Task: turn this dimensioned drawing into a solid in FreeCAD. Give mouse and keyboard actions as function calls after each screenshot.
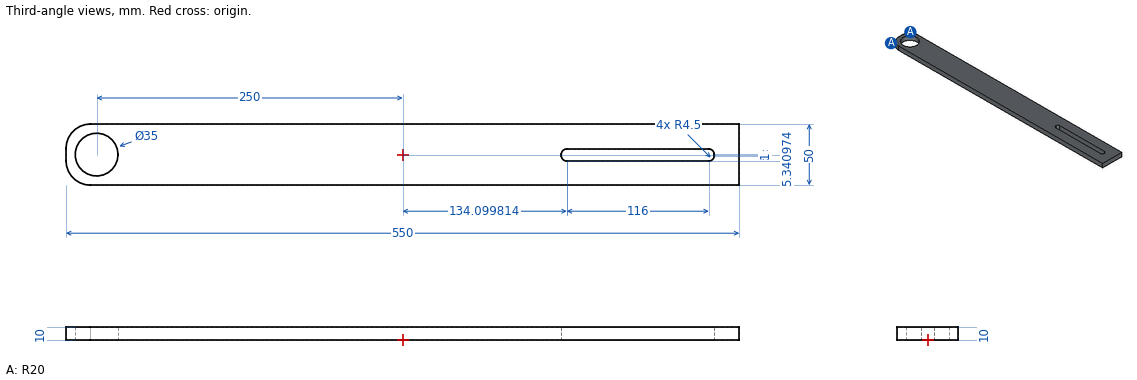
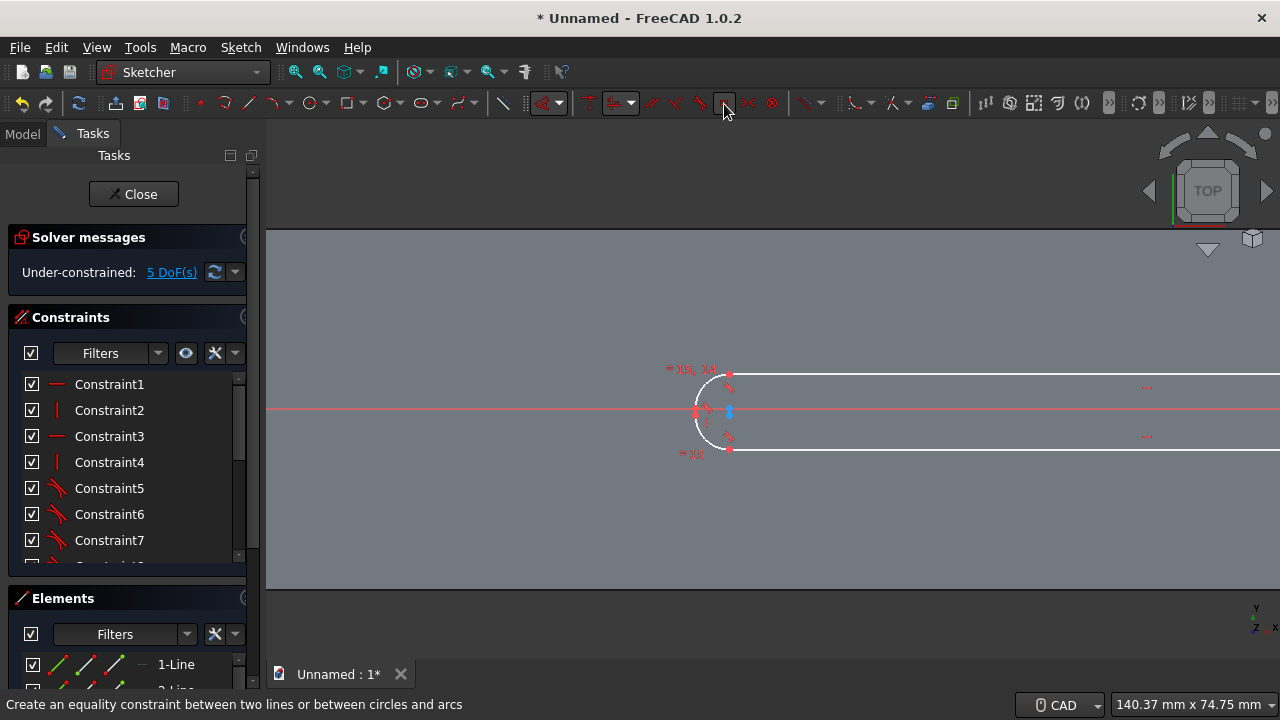
scroll(715, 379, down, 6)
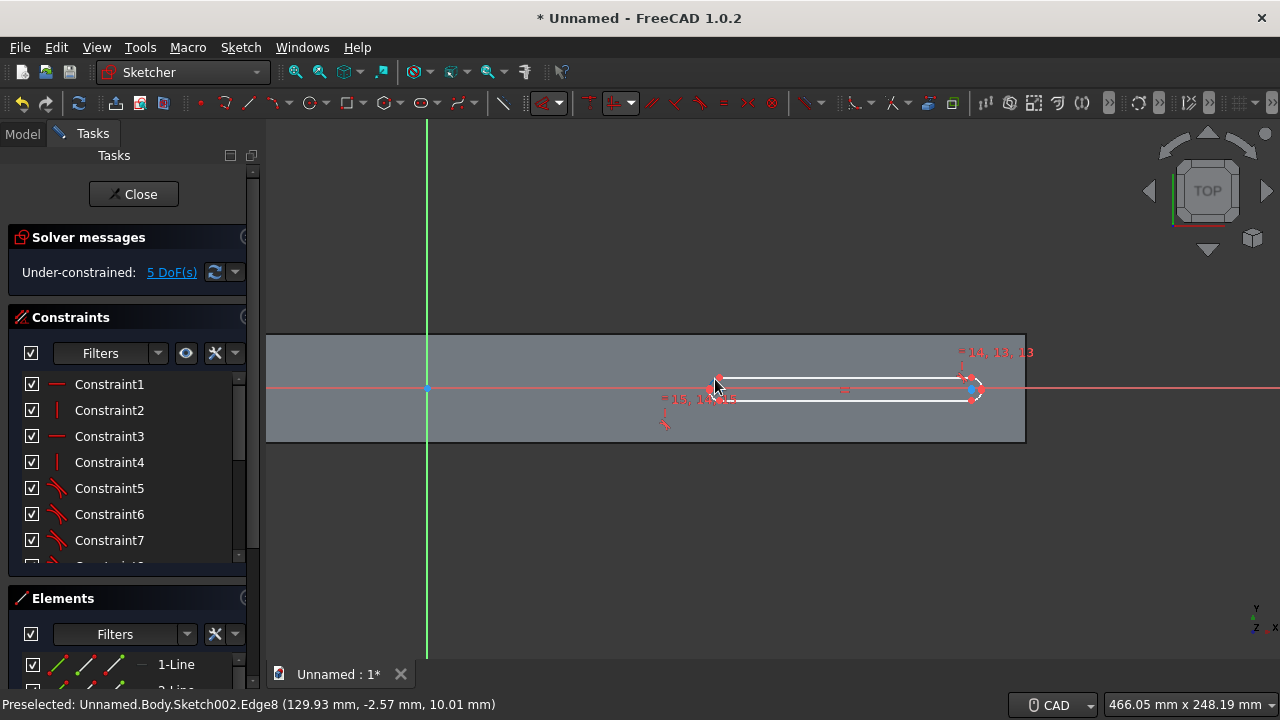
scroll(976, 400, up, 7)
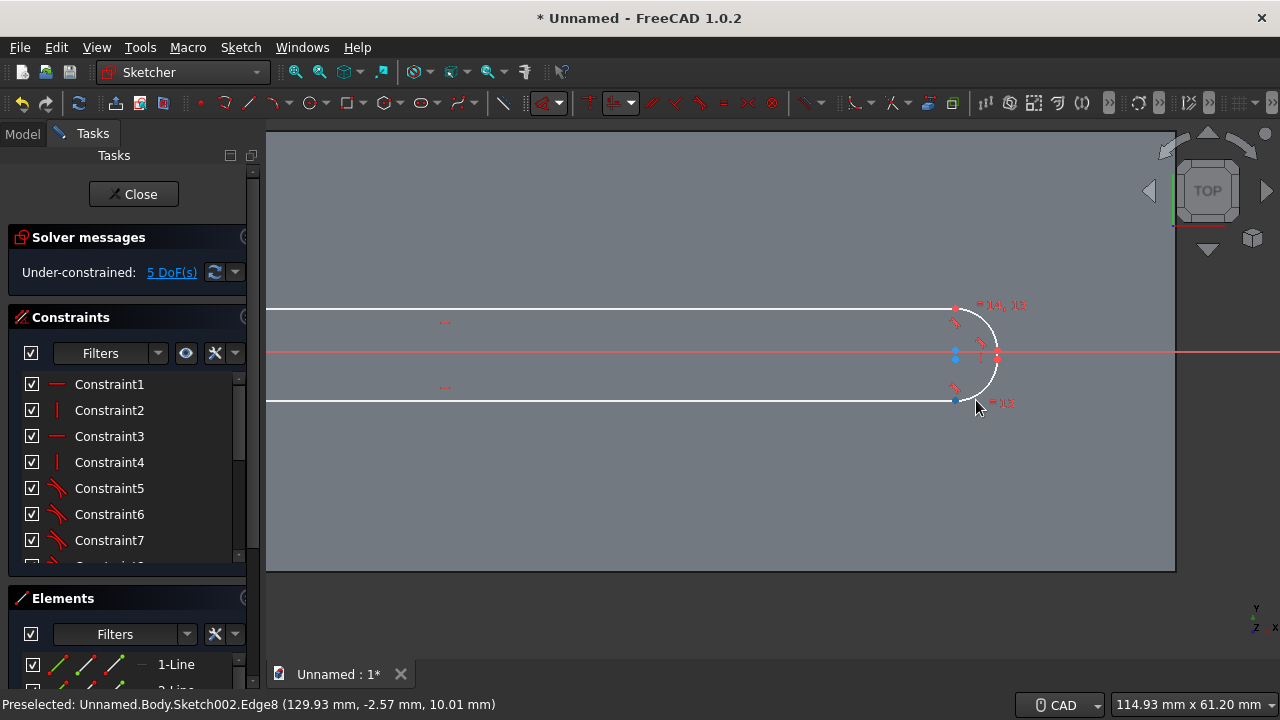
click(974, 396)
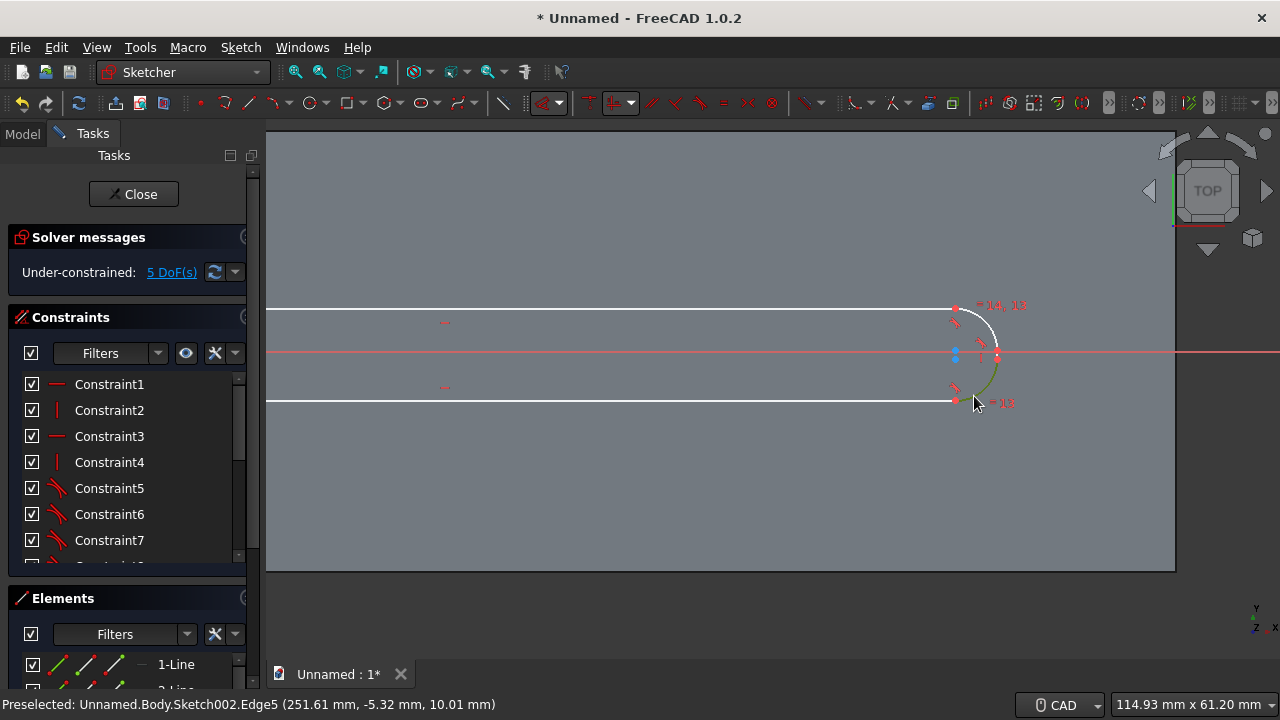
key(k)
key(r)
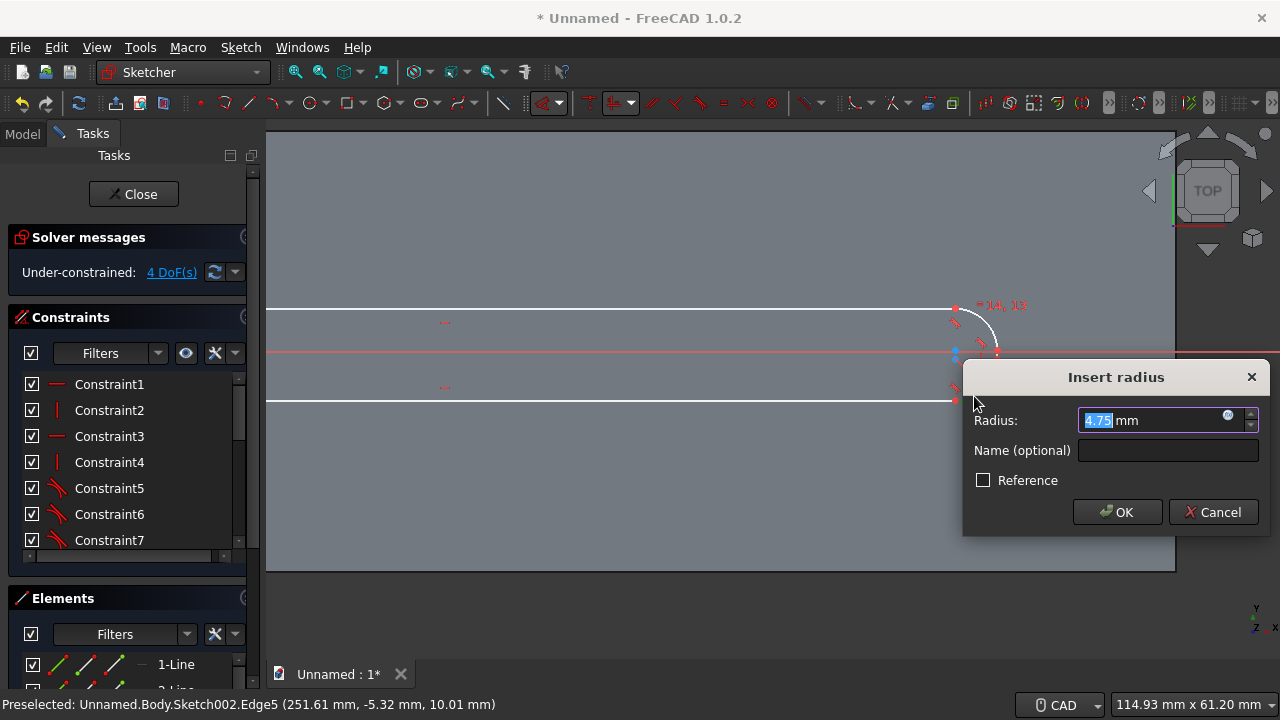
text(4.5)
key(Return)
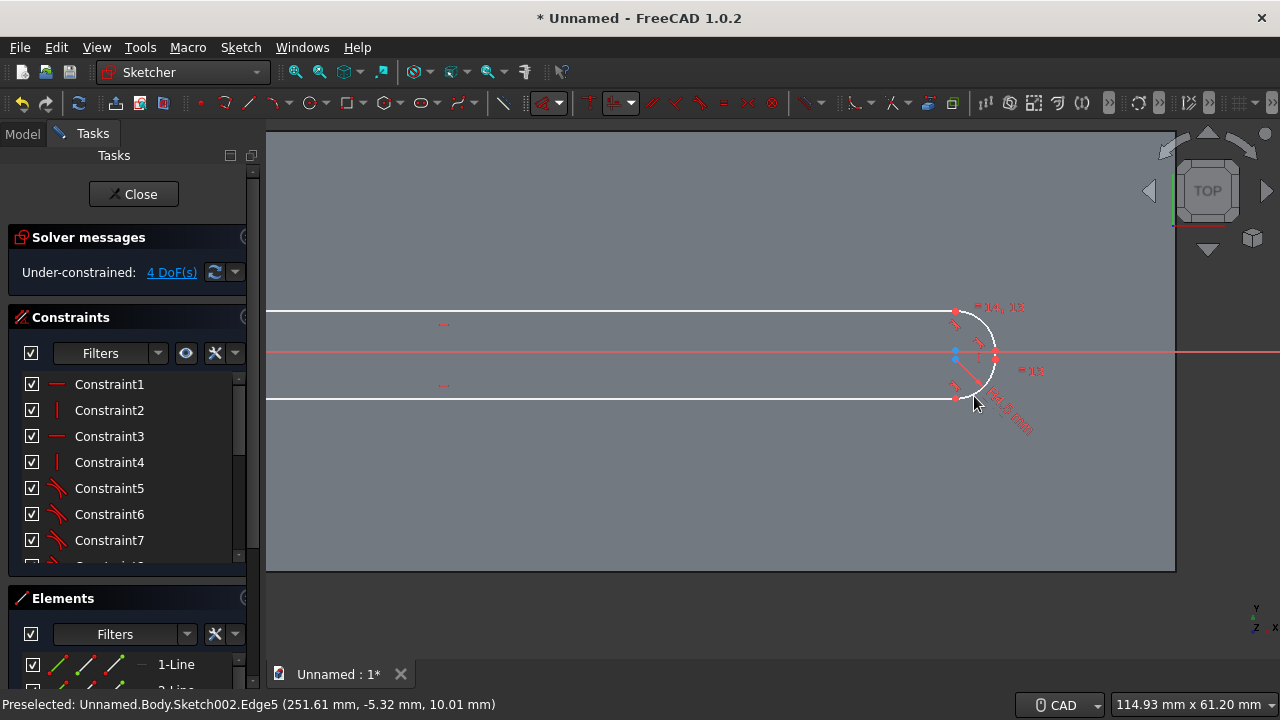
scroll(995, 355, up, 8)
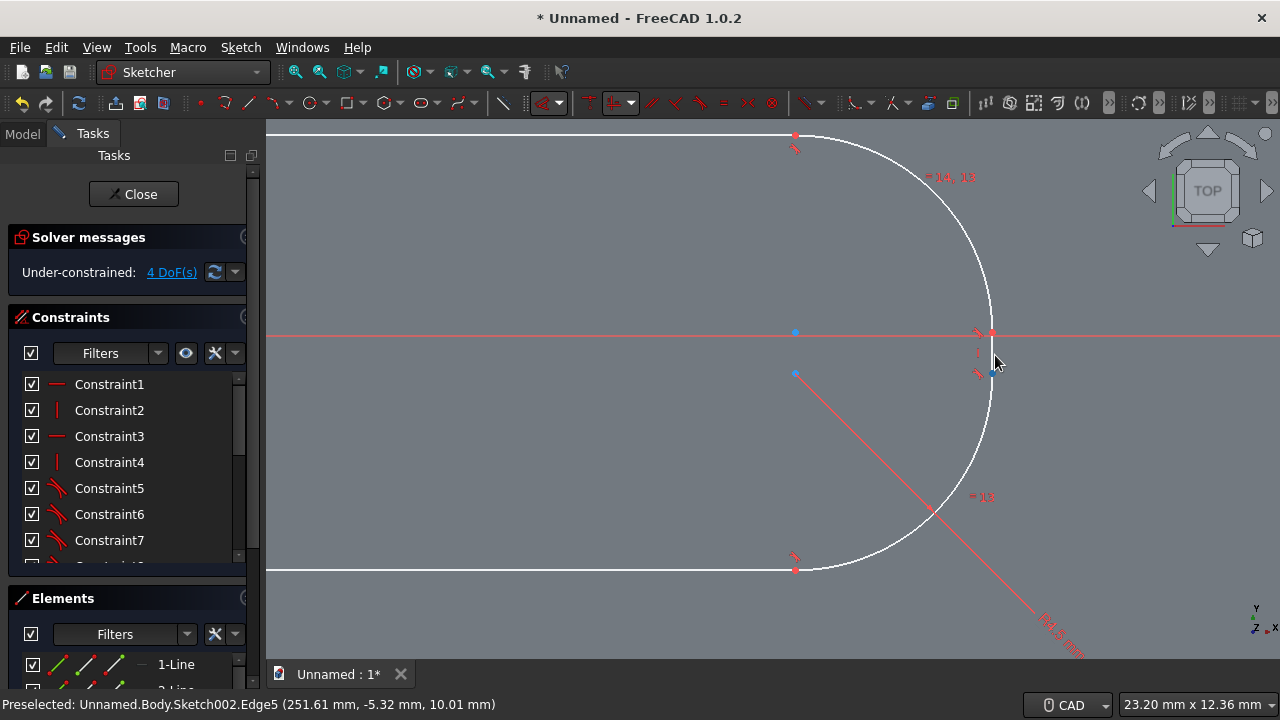
click(992, 353)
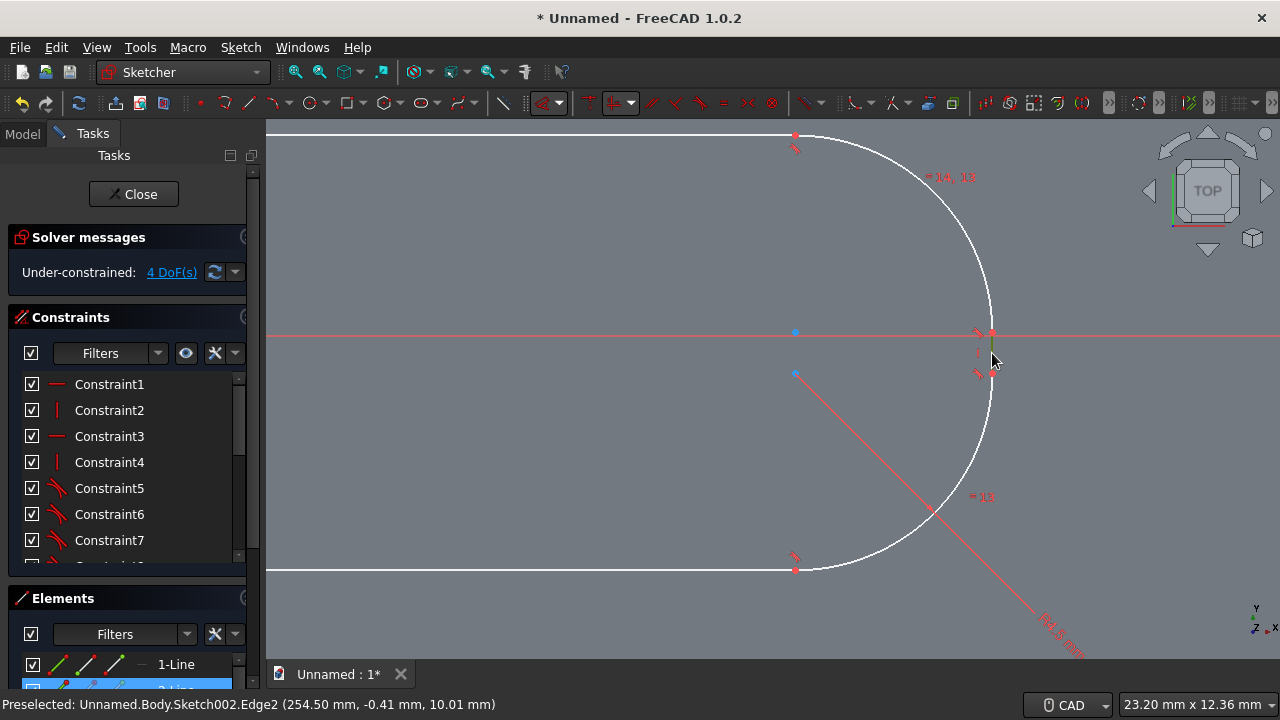
click(562, 104)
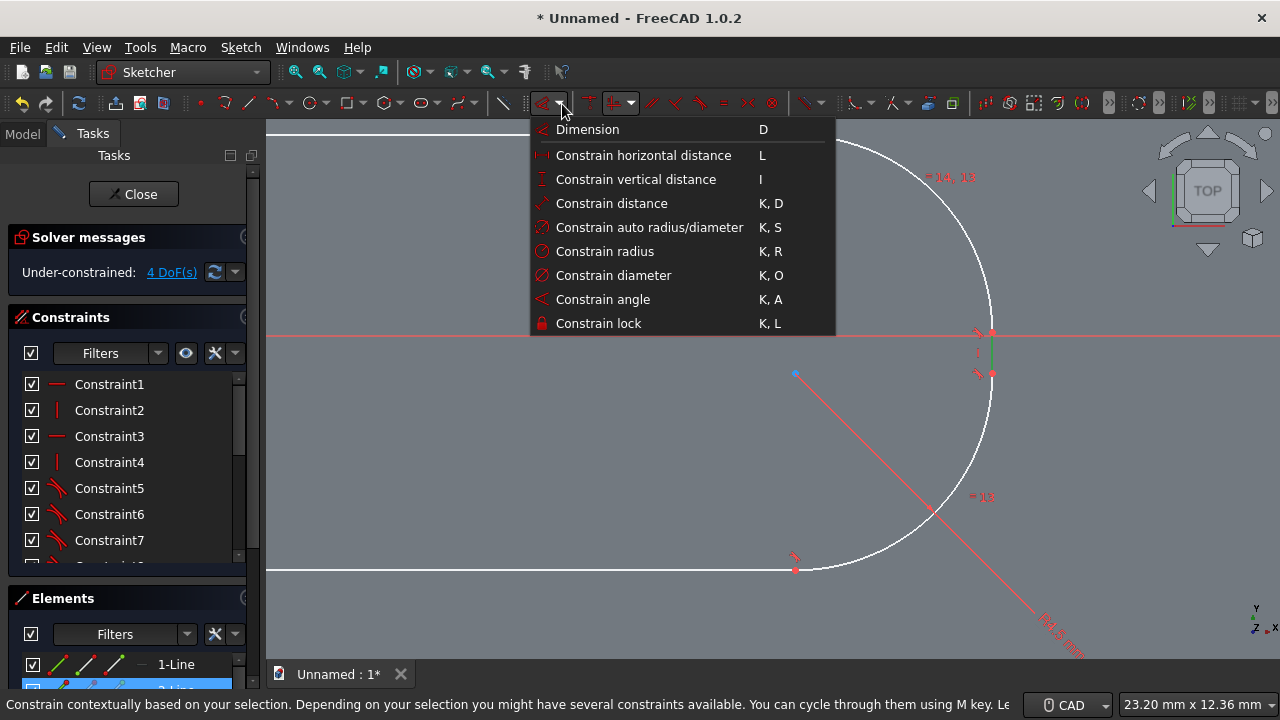
click(683, 179)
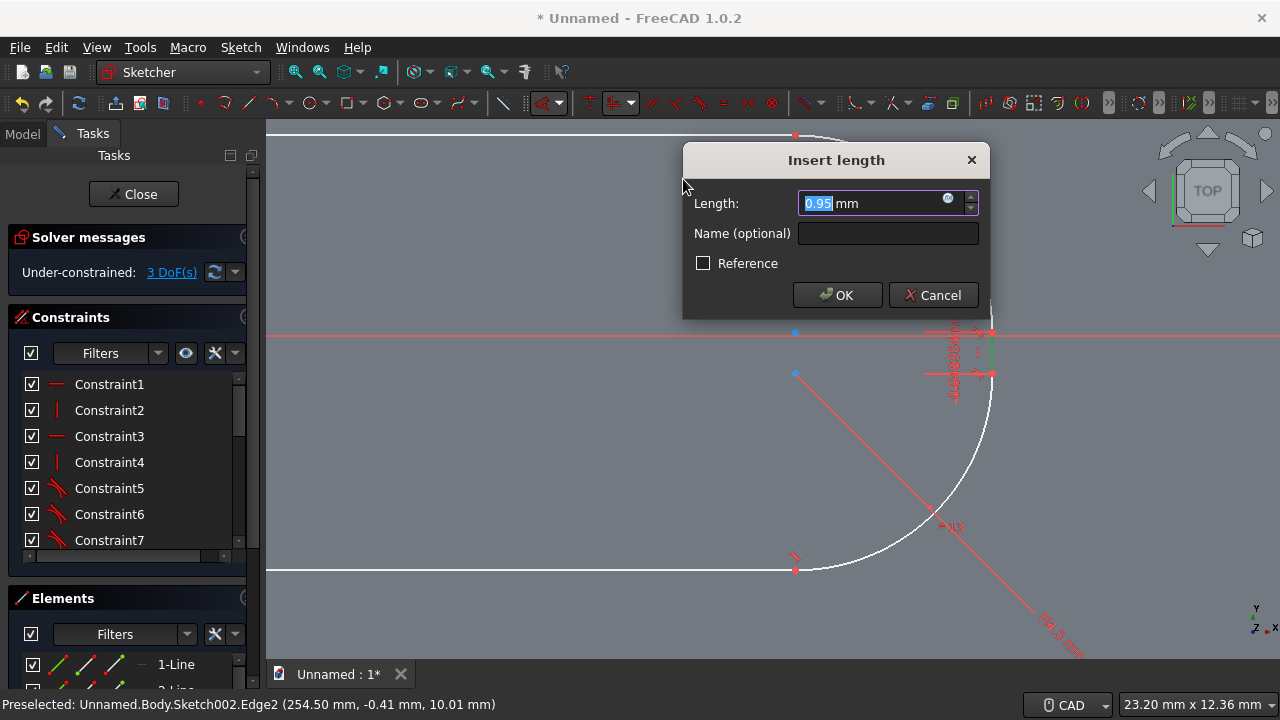
text(1)
key(Return)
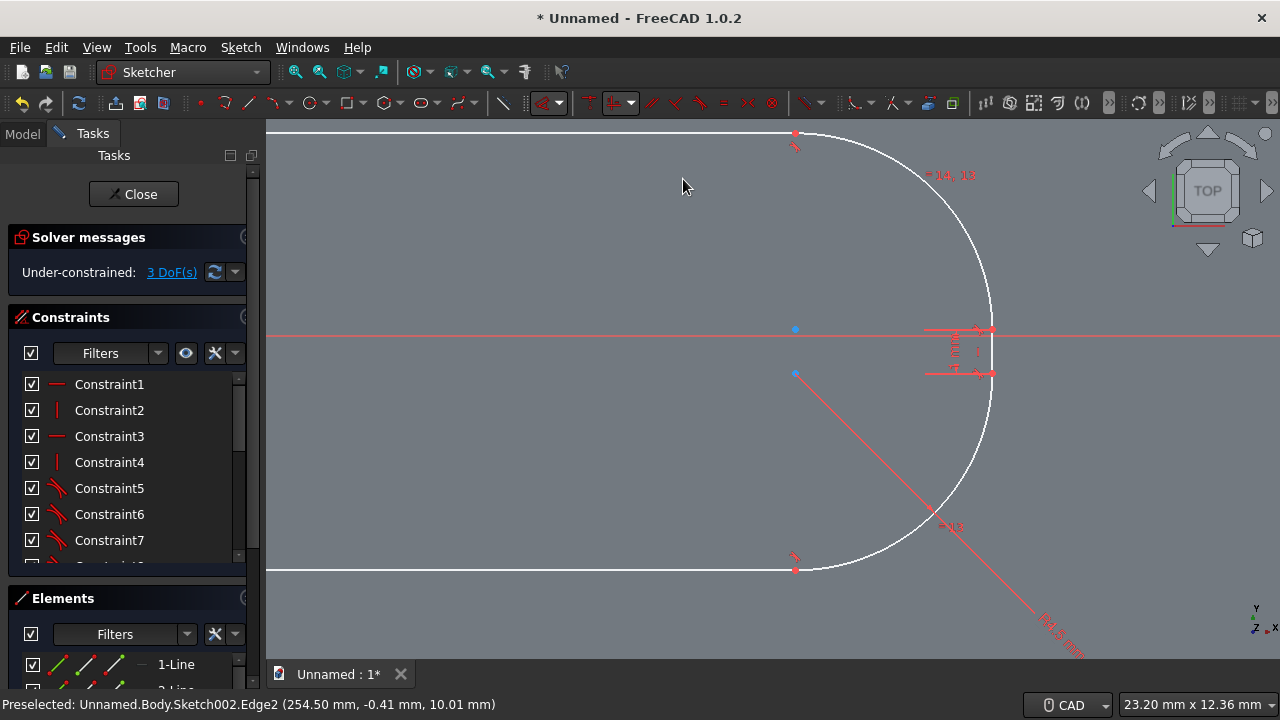
scroll(981, 391, down, 15)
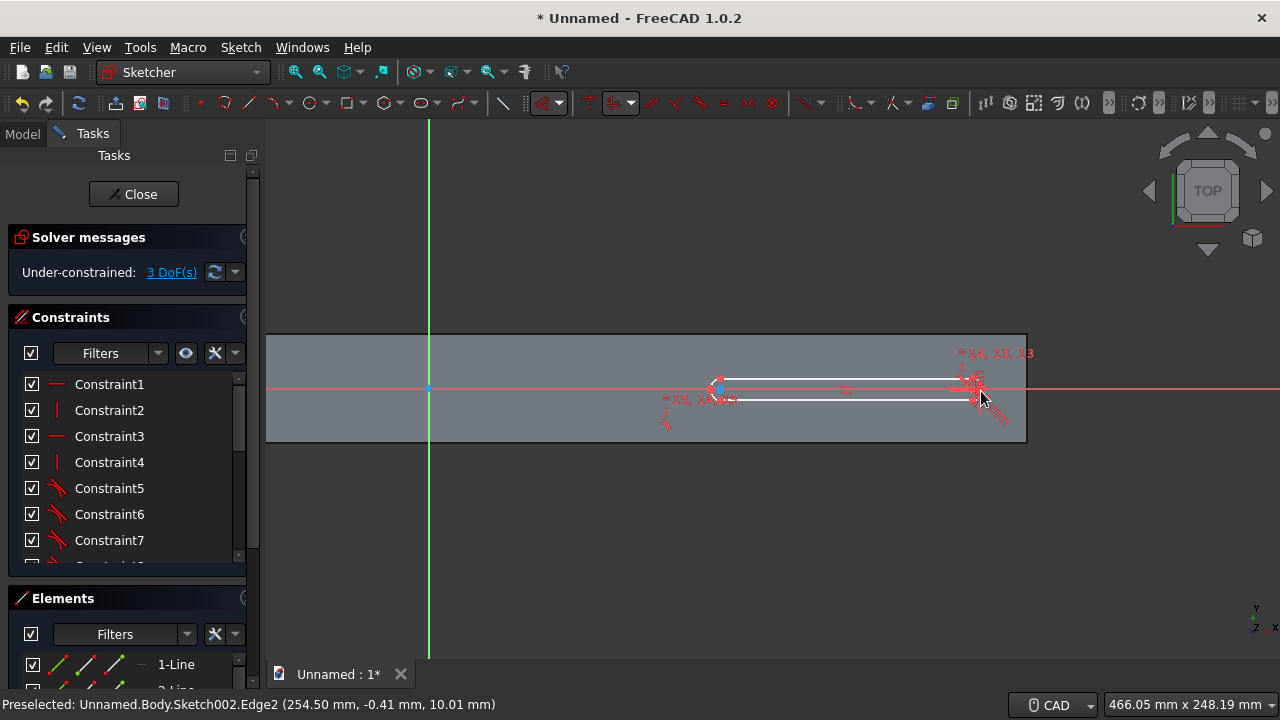
click(796, 400)